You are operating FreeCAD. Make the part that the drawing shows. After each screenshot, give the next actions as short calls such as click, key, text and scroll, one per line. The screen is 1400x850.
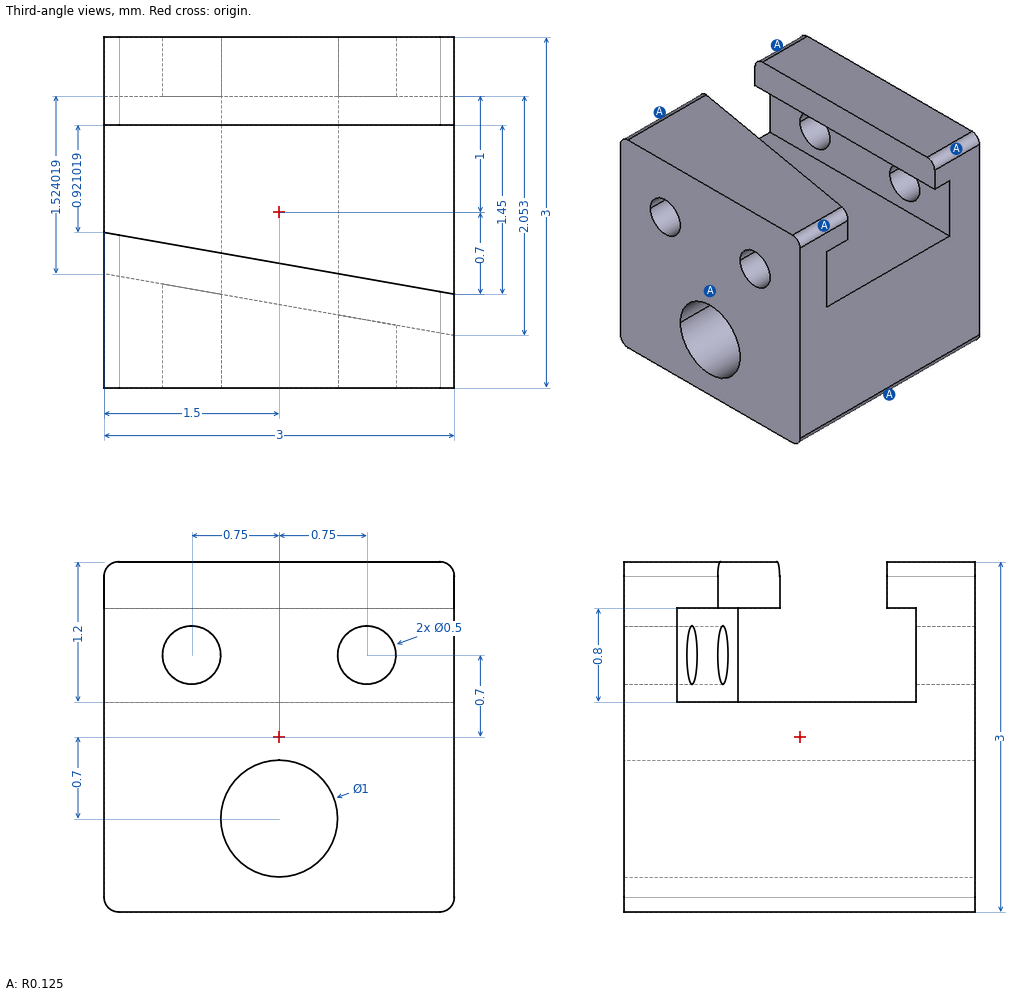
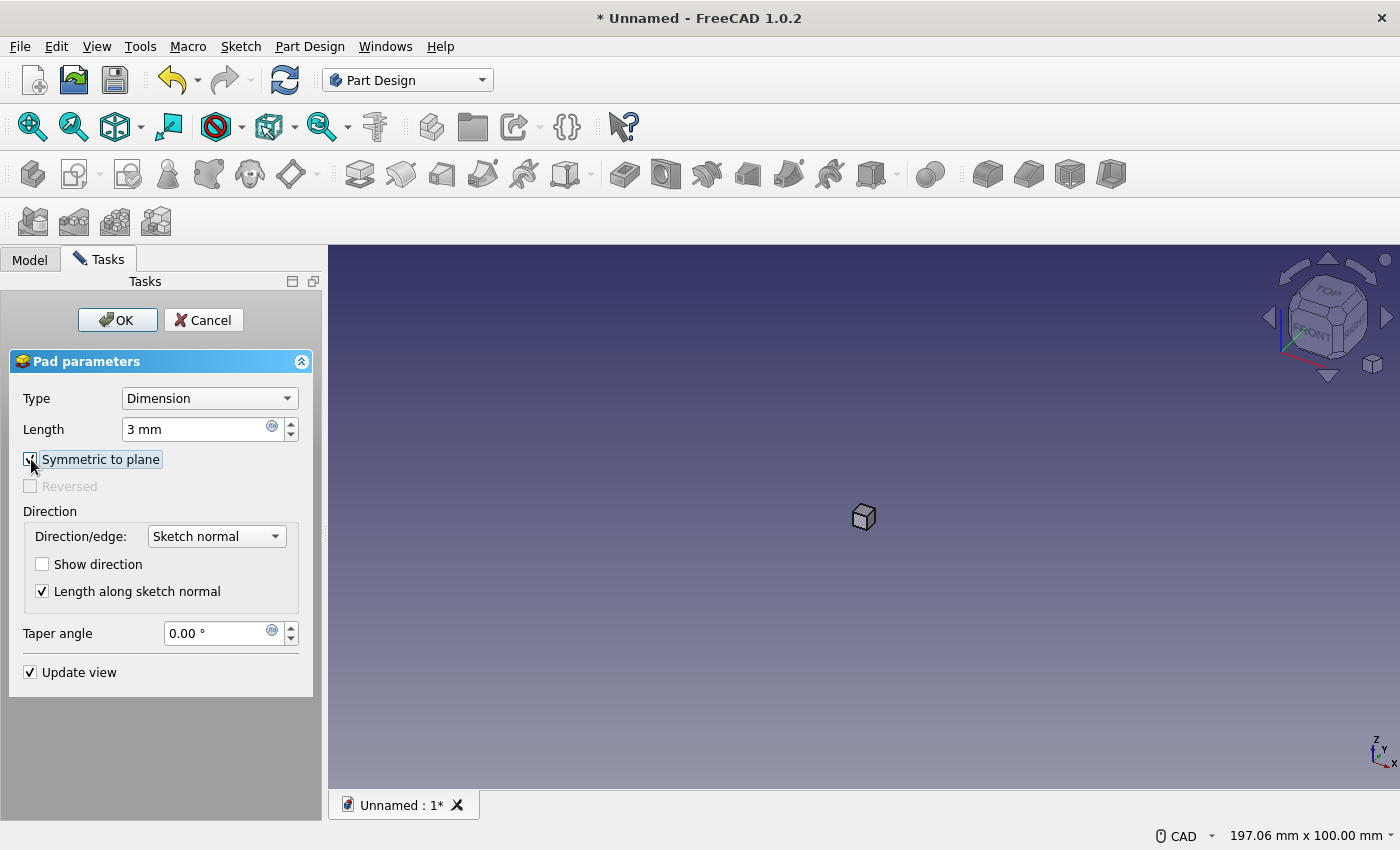
click(118, 320)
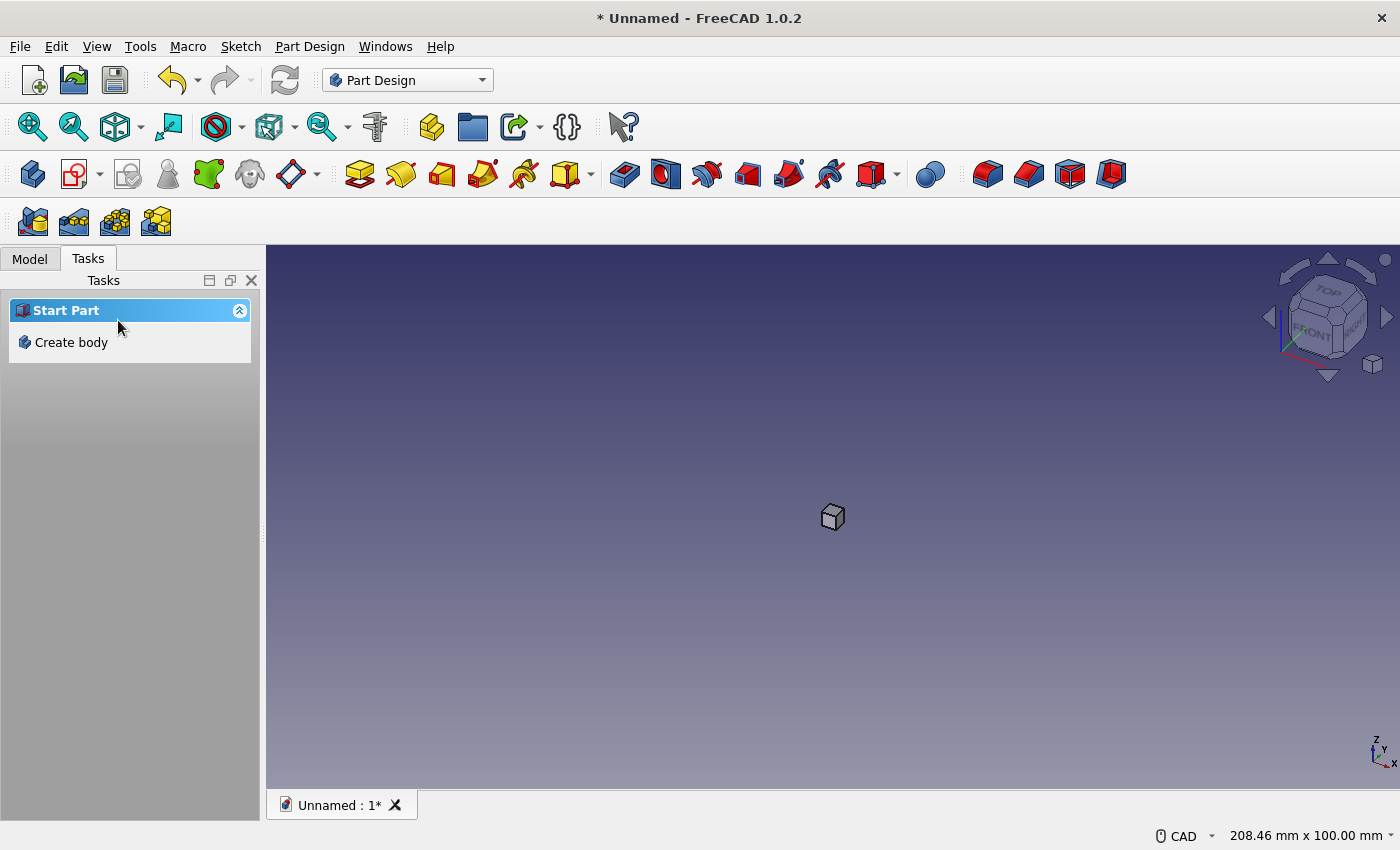
key(v)
key(f)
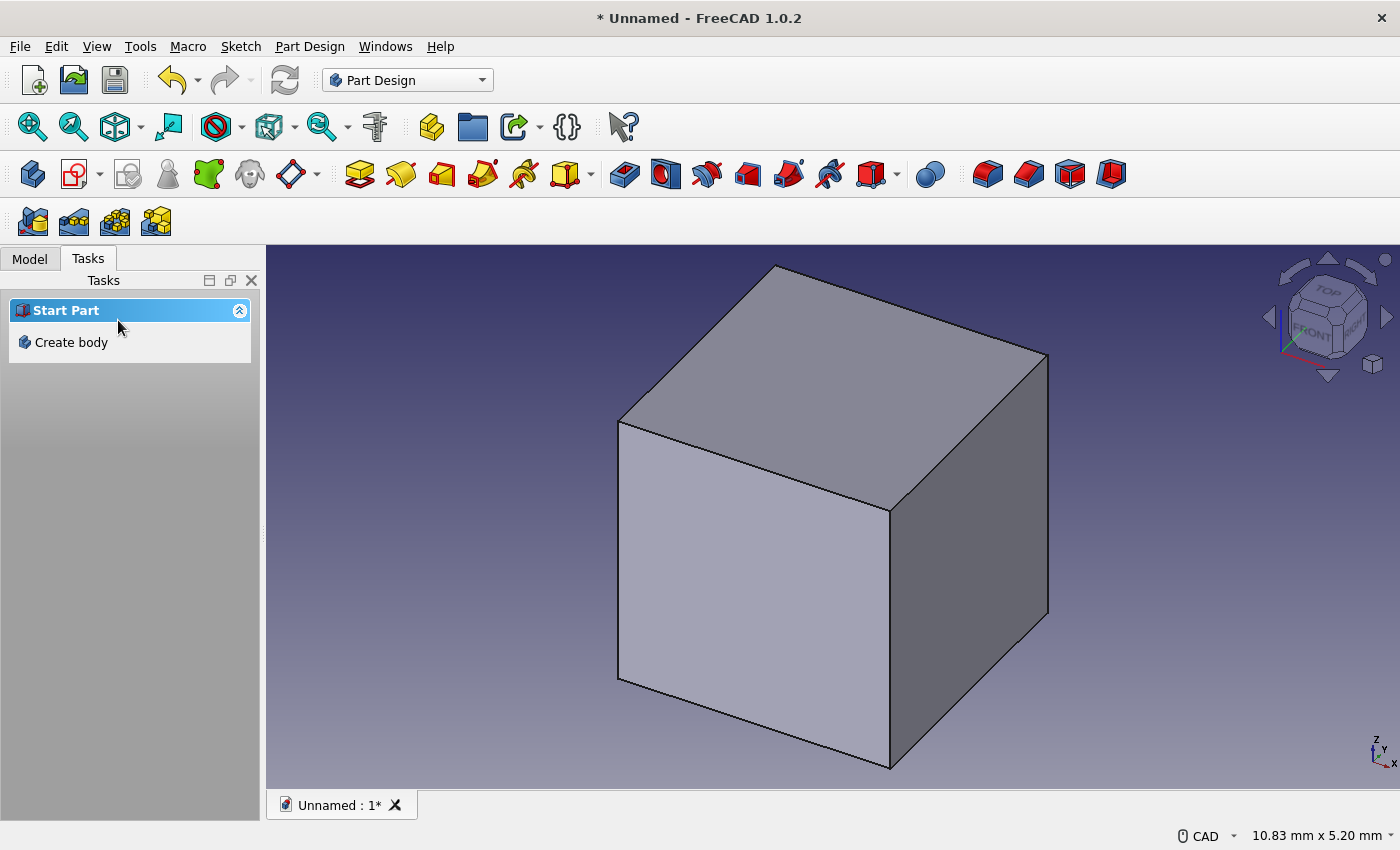
click(833, 387)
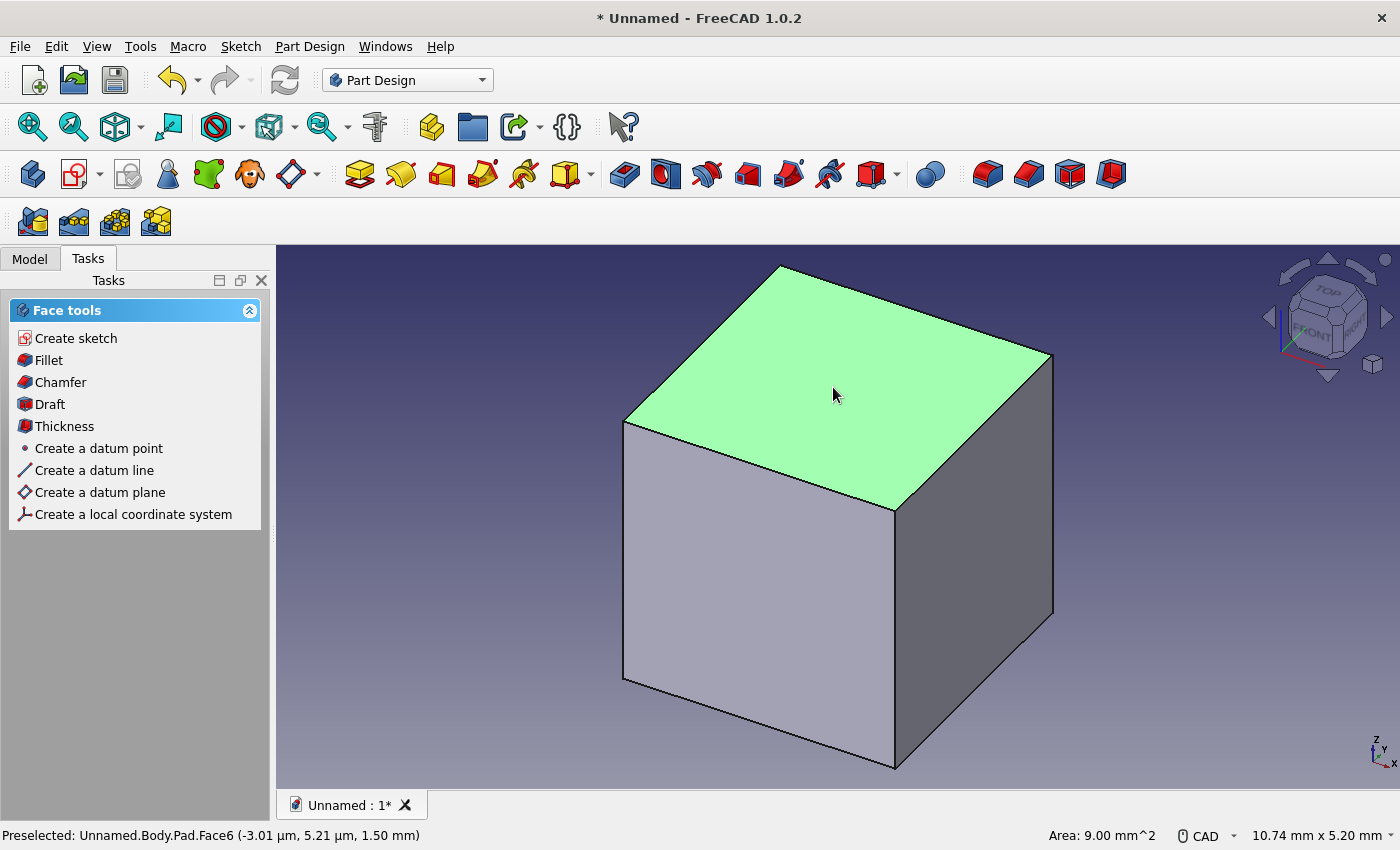
click(74, 174)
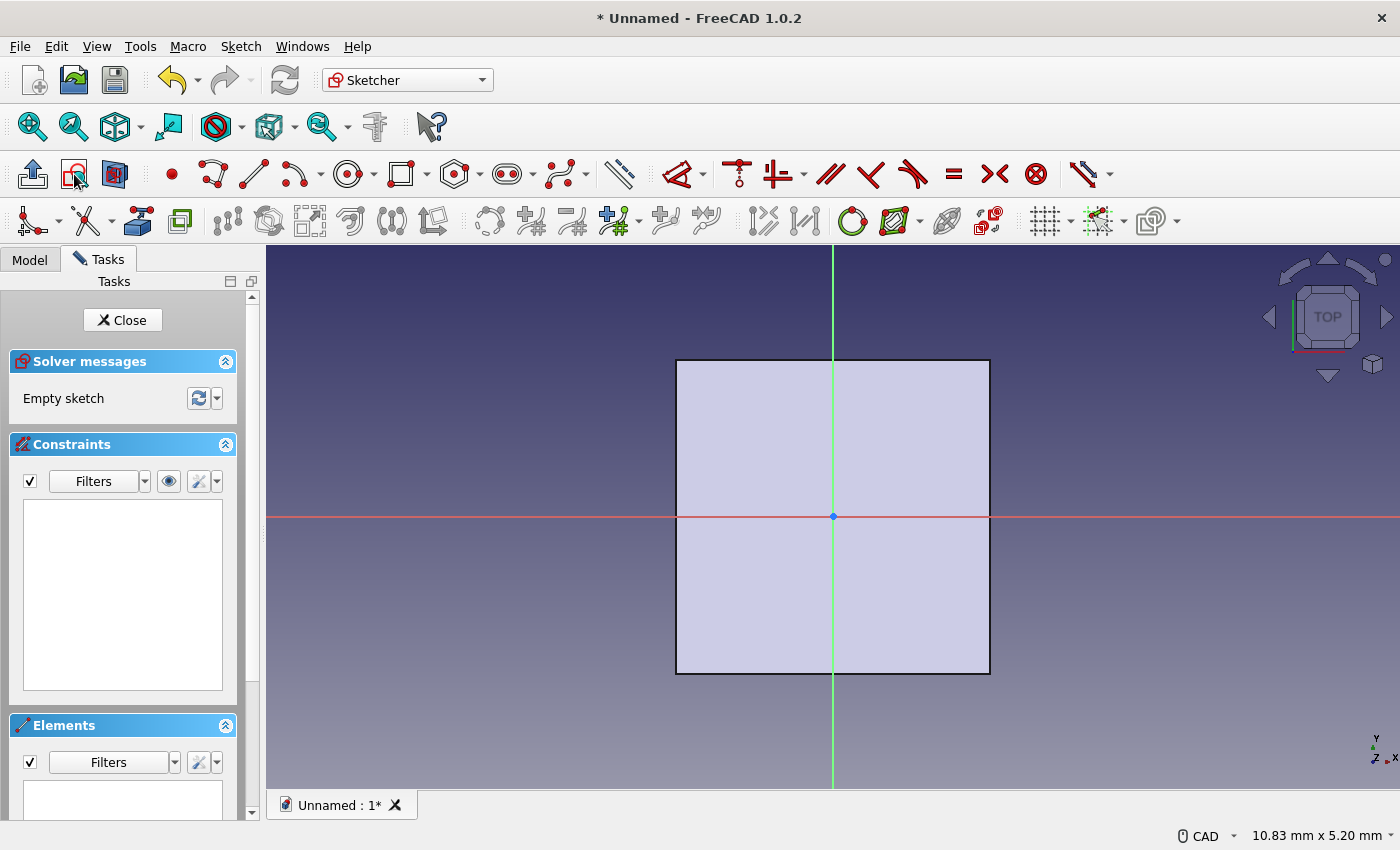
scroll(889, 512, up, 4)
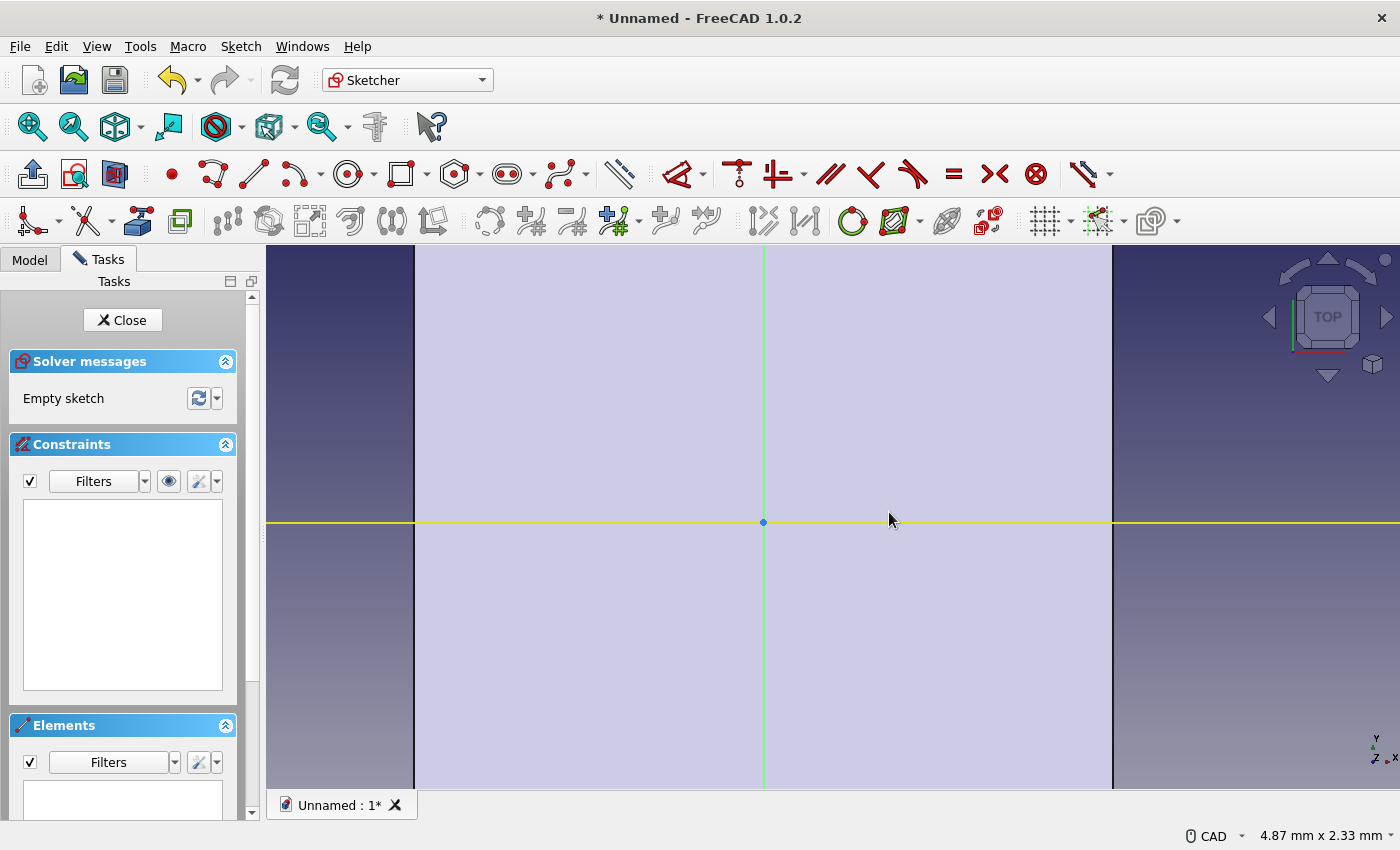
key(g)
key(m)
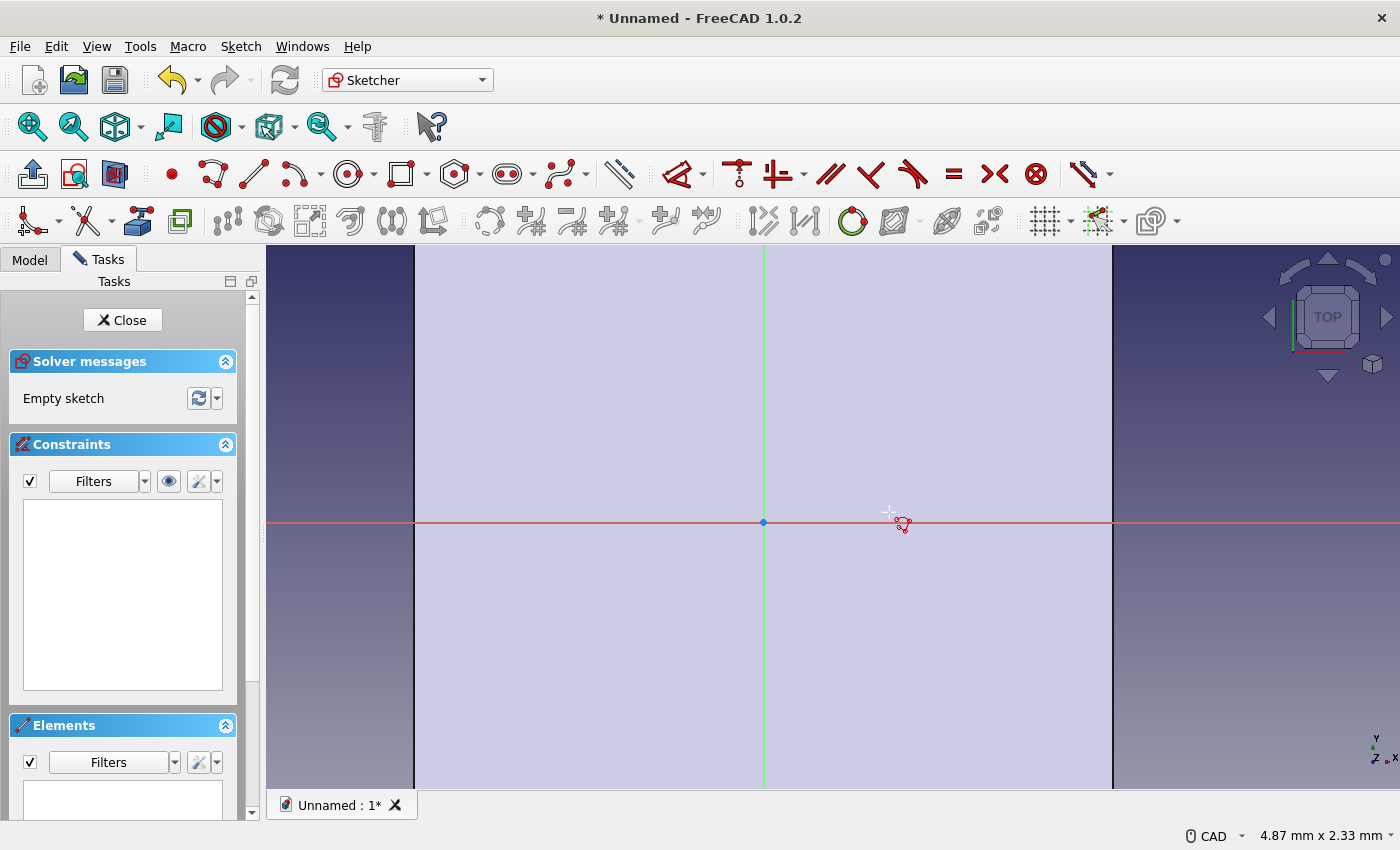
click(414, 562)
click(1113, 686)
click(1113, 348)
click(414, 348)
click(414, 563)
key(Escape)
key(Escape)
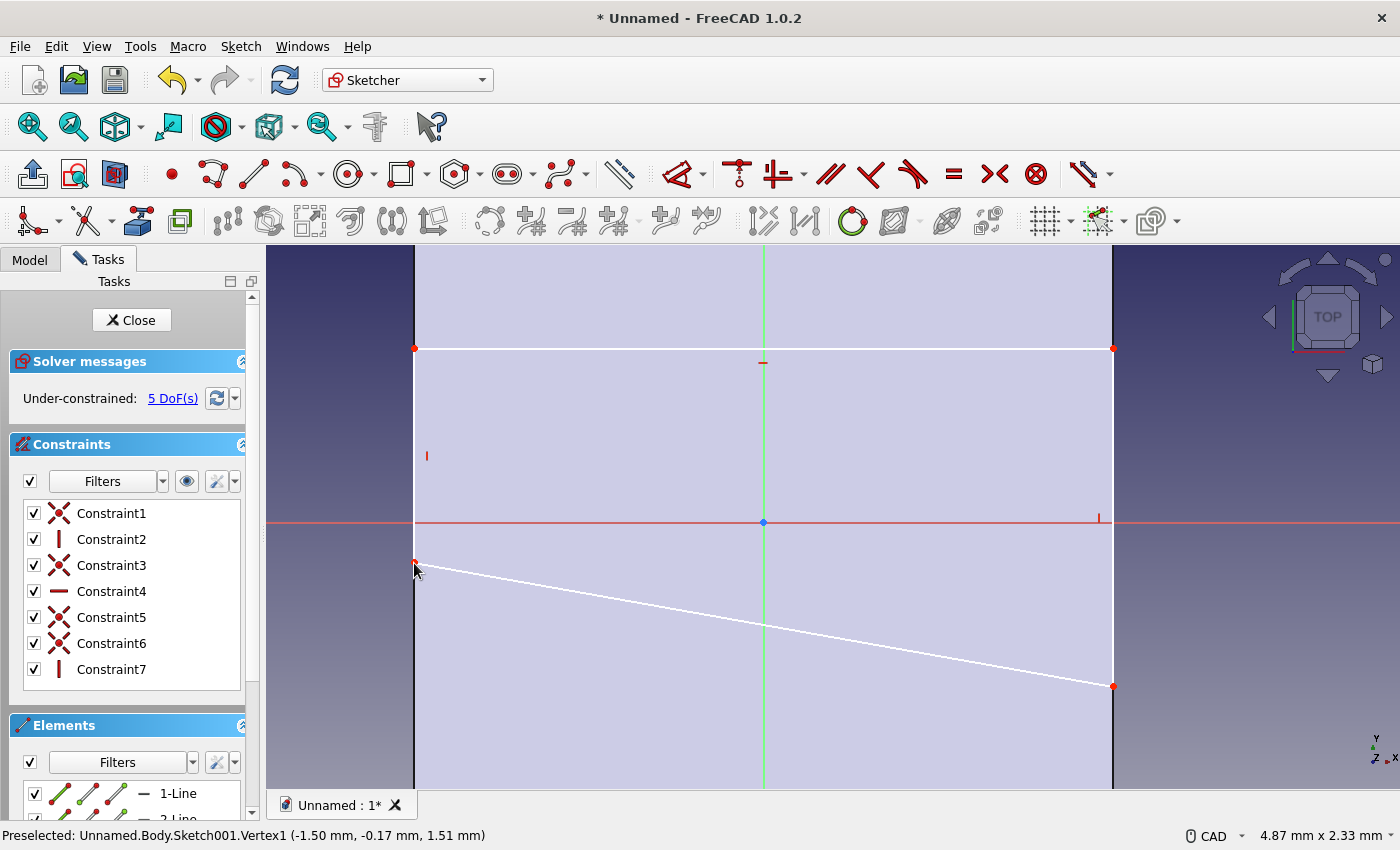
key(d)